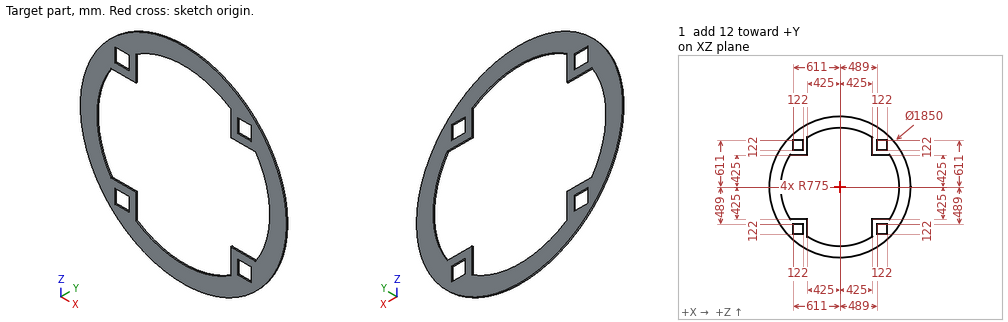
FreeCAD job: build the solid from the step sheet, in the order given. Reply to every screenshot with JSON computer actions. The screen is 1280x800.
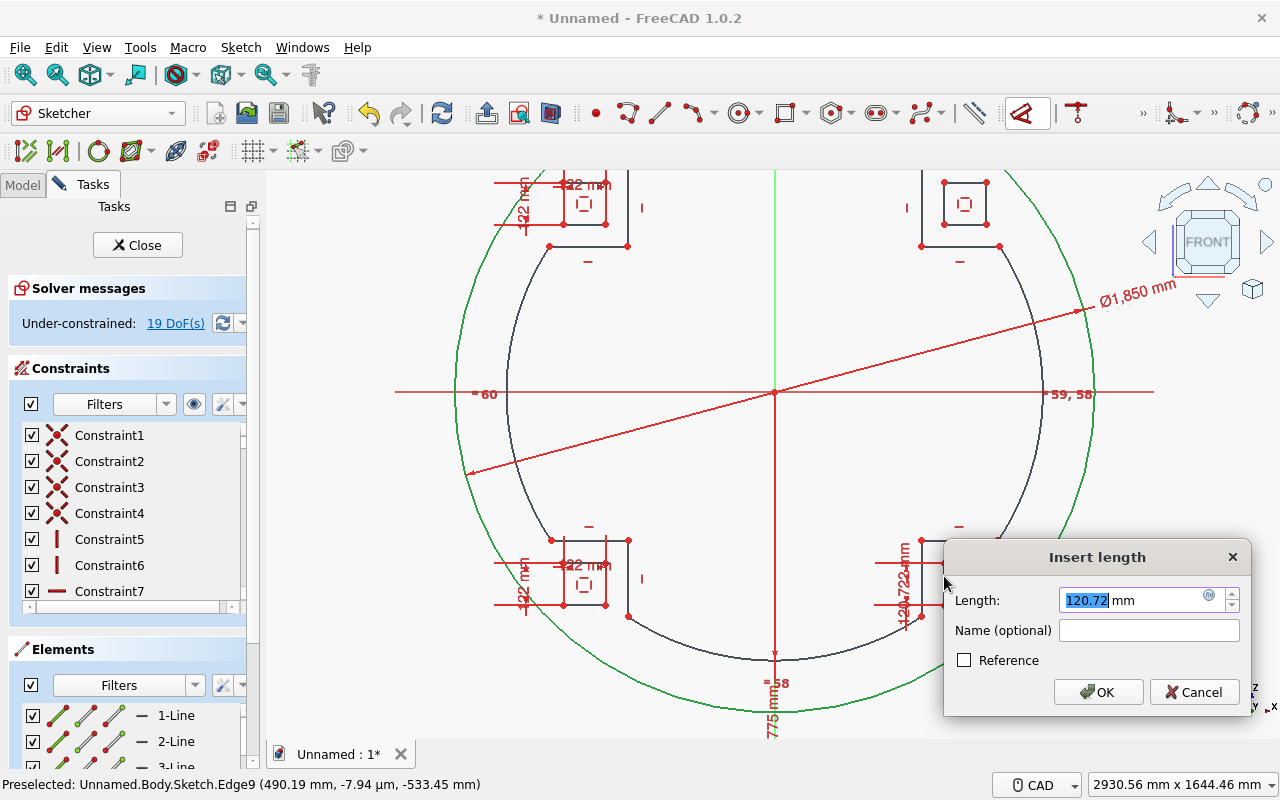
{"action": "type", "text": "122"}
{"action": "key", "text": "Return"}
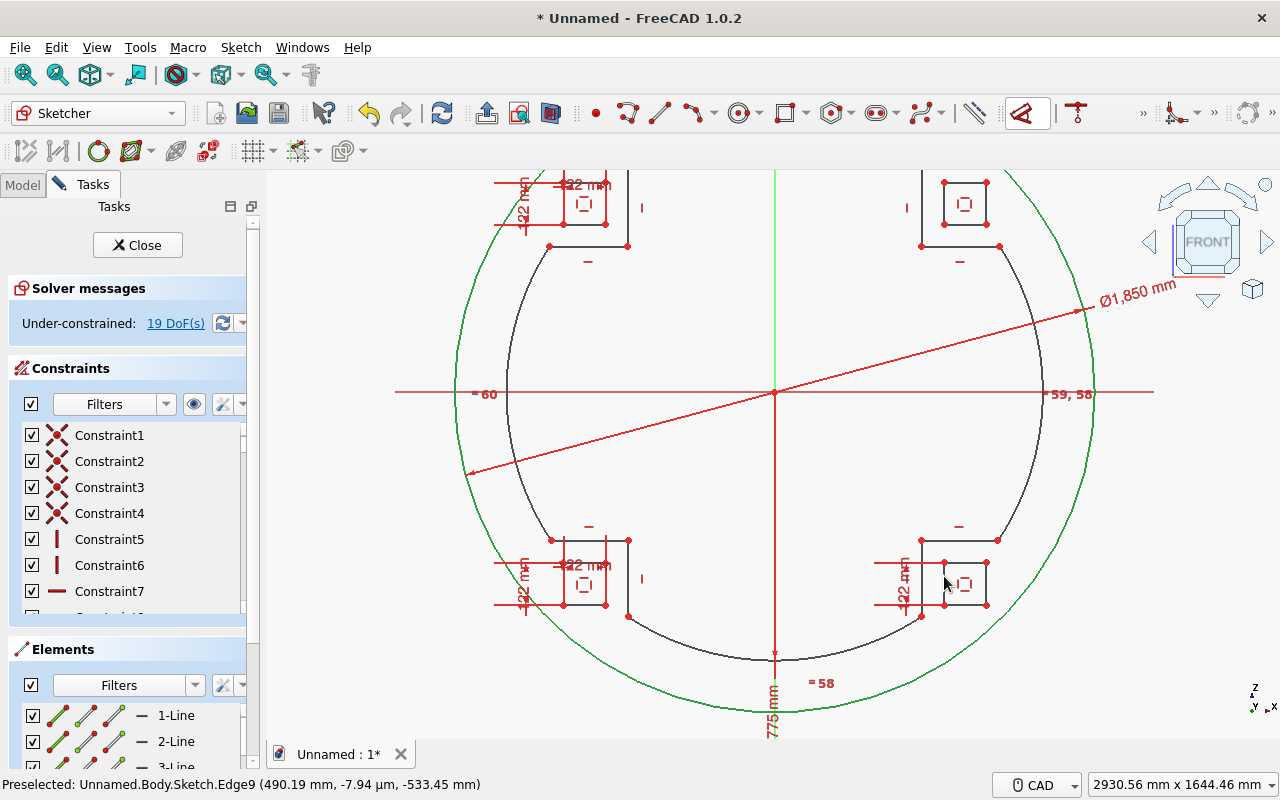
{"action": "left_click", "coordinate": [957, 605]}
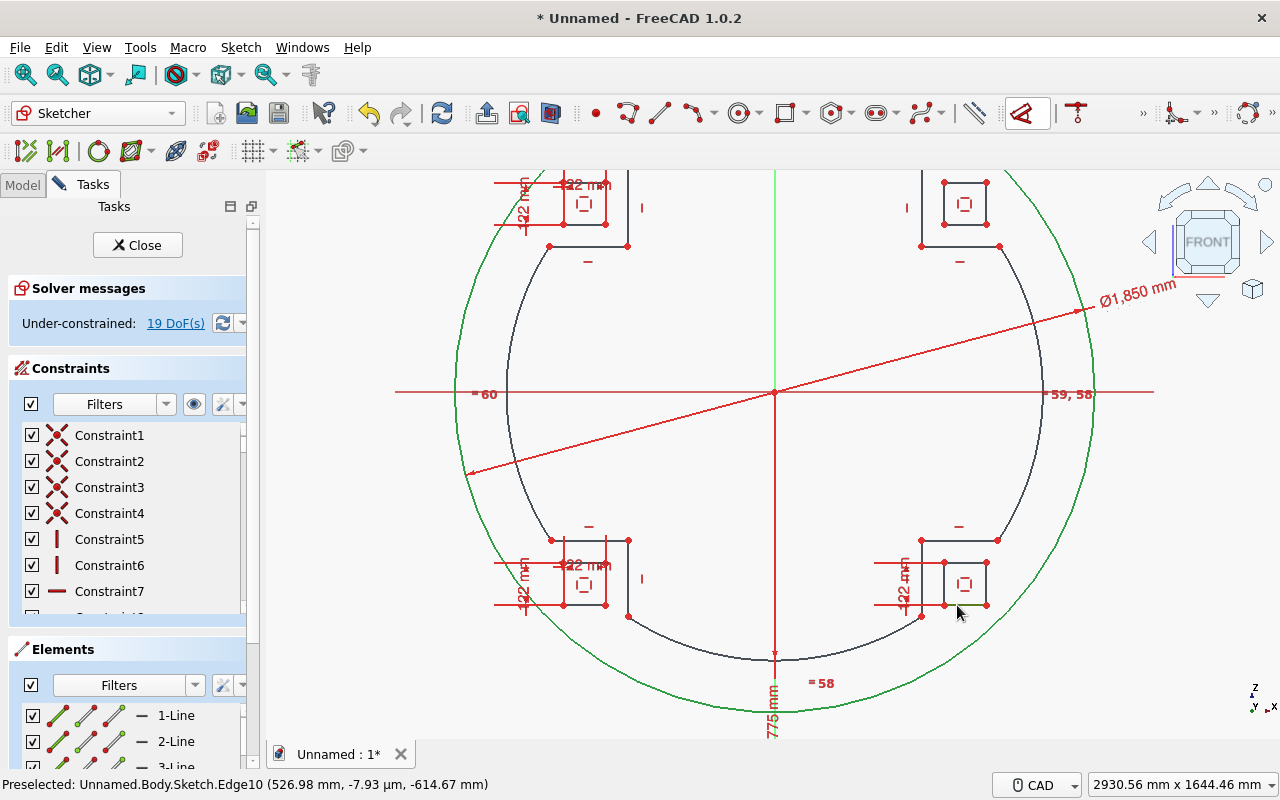
{"action": "left_click", "coordinate": [1044, 114]}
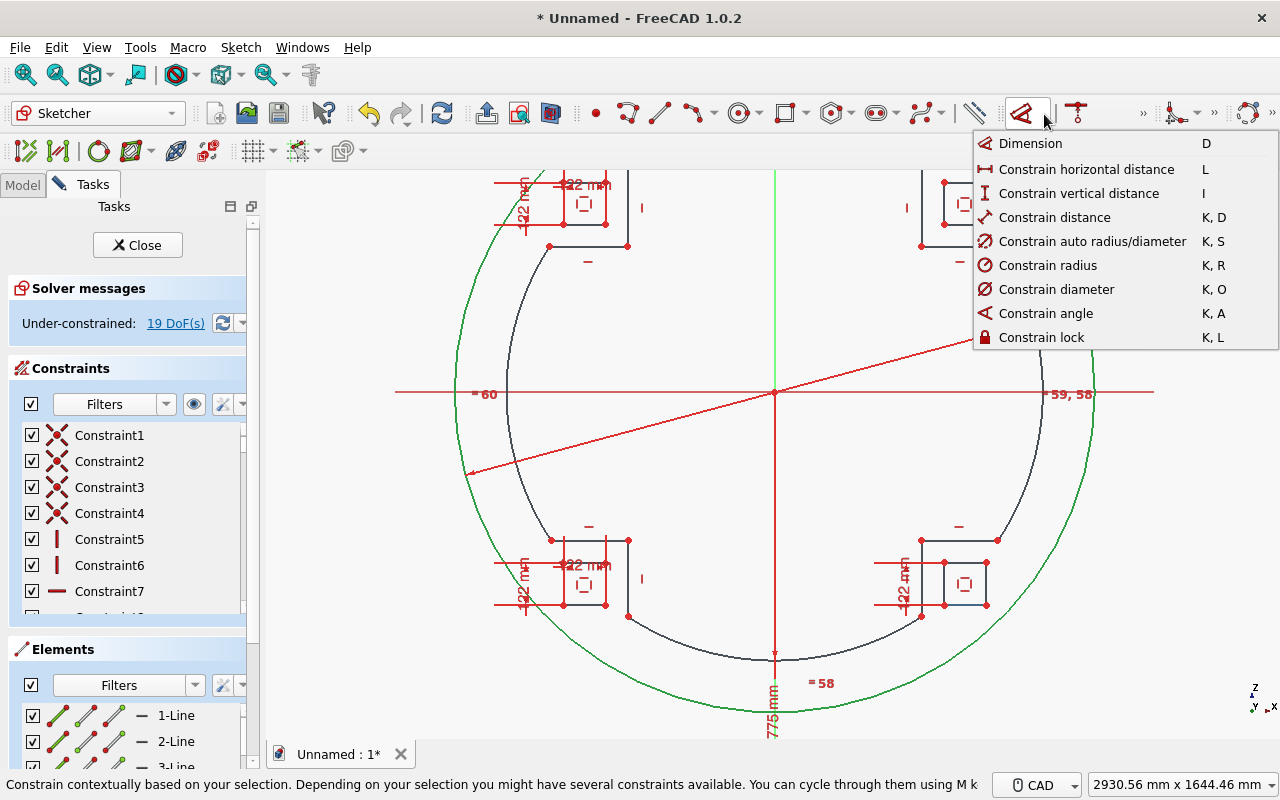
{"action": "left_click", "coordinate": [1126, 169]}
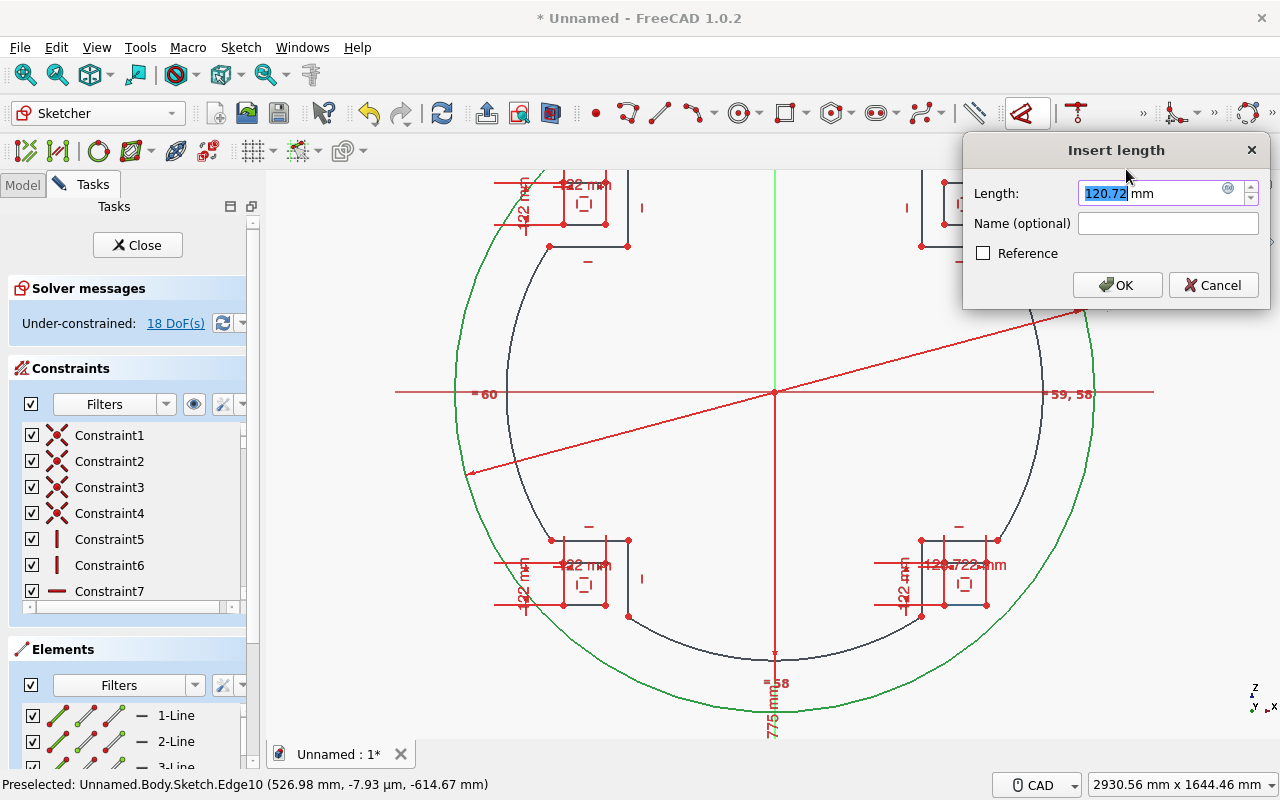
{"action": "type", "text": "122"}
{"action": "key", "text": "Return"}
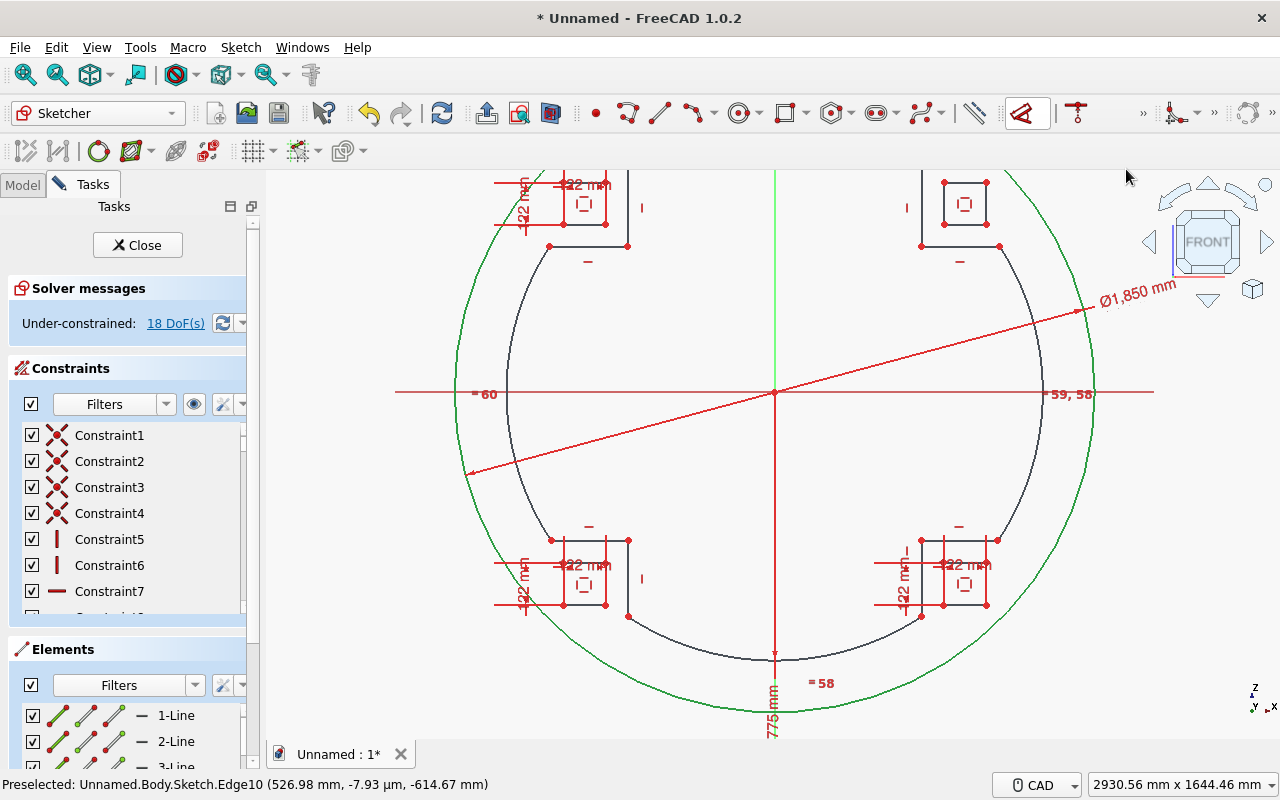
{"action": "left_click", "coordinate": [944, 212]}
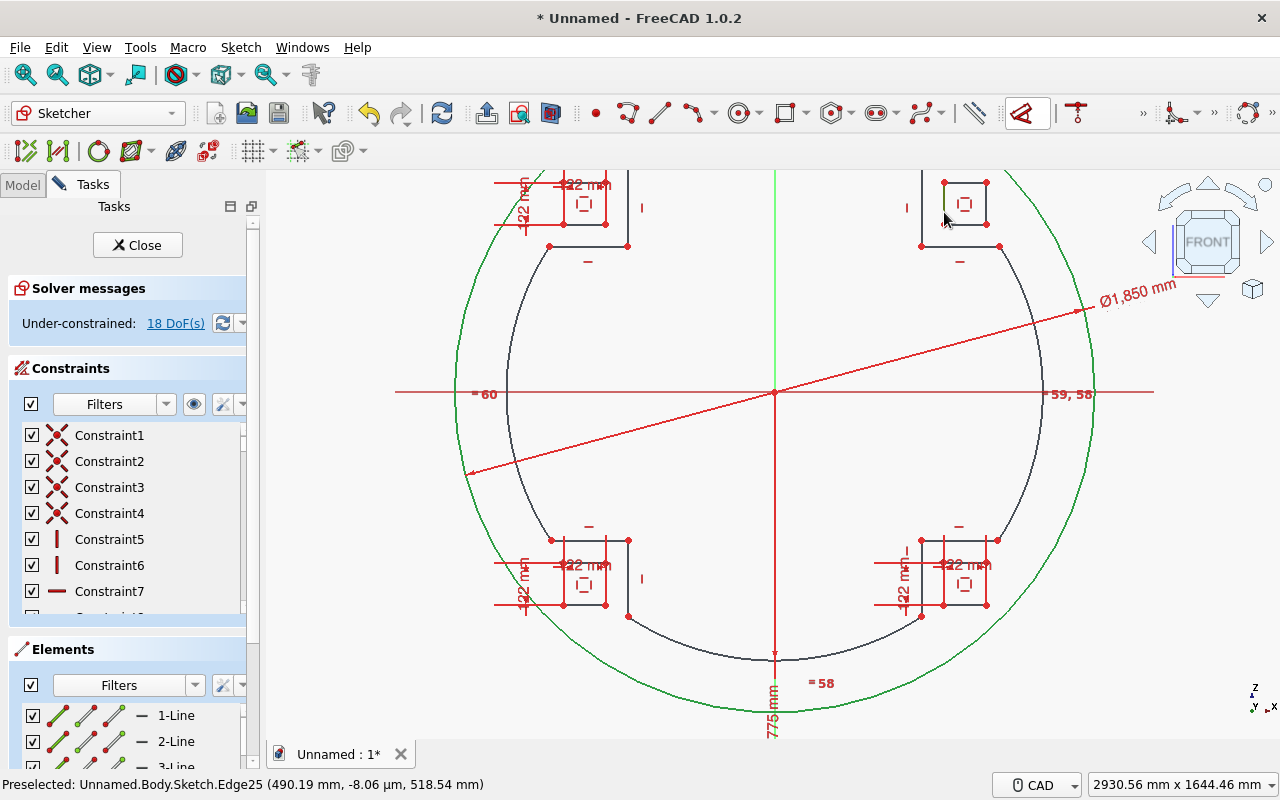
{"action": "key", "text": "i"}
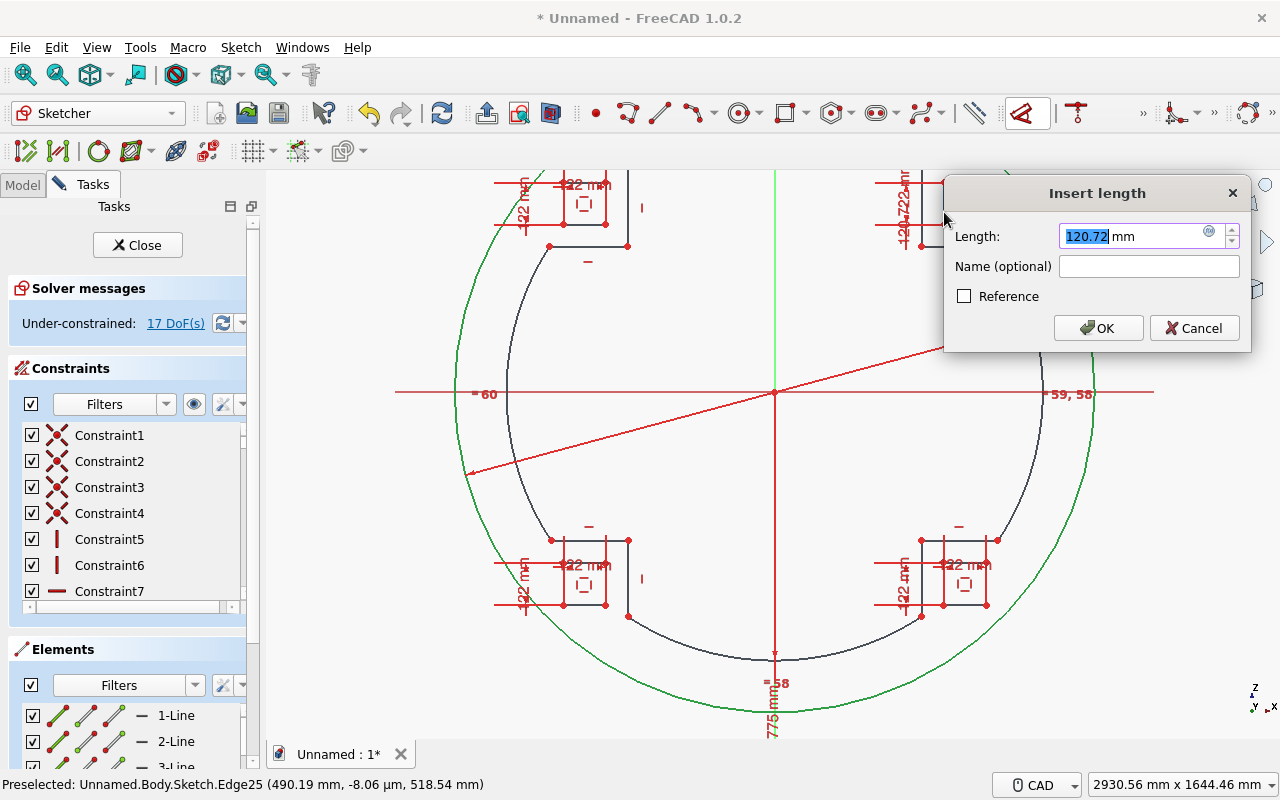
{"action": "type", "text": "122"}
{"action": "key", "text": "Return"}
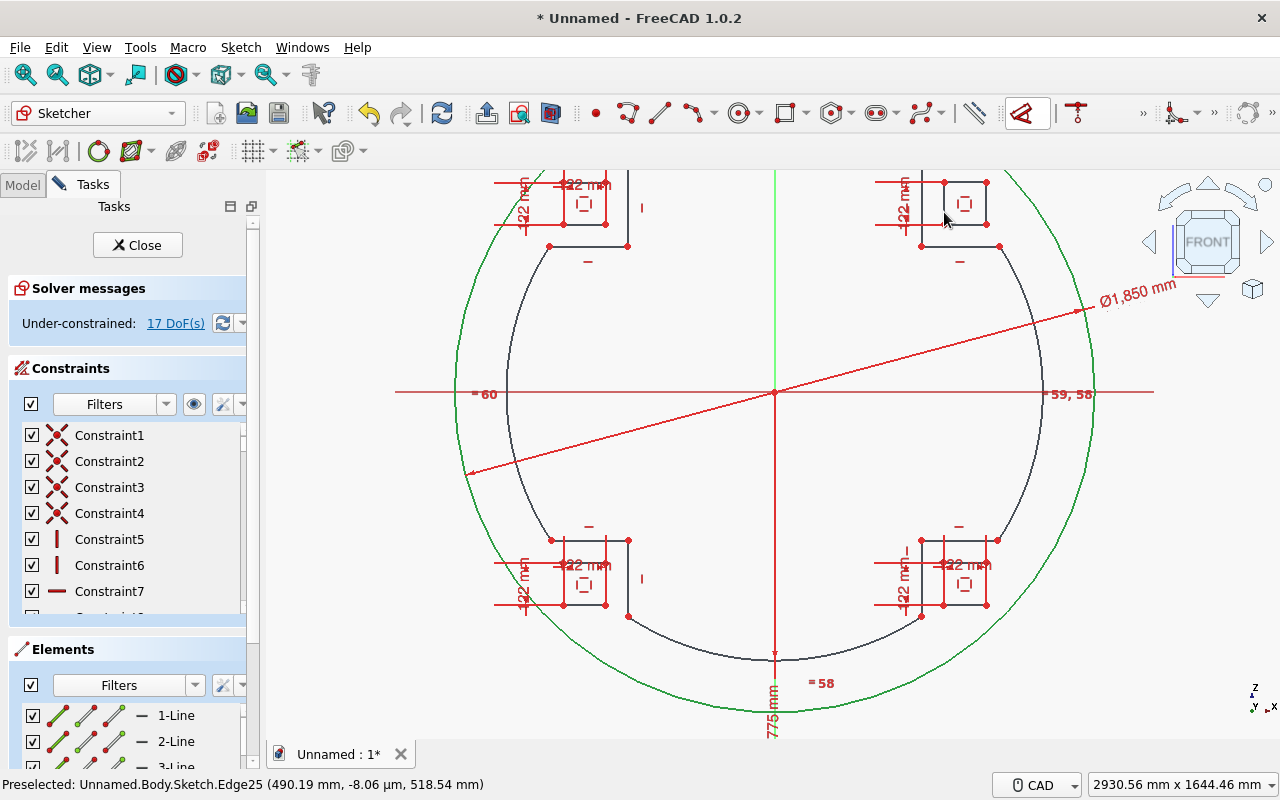
{"action": "left_click", "coordinate": [957, 225]}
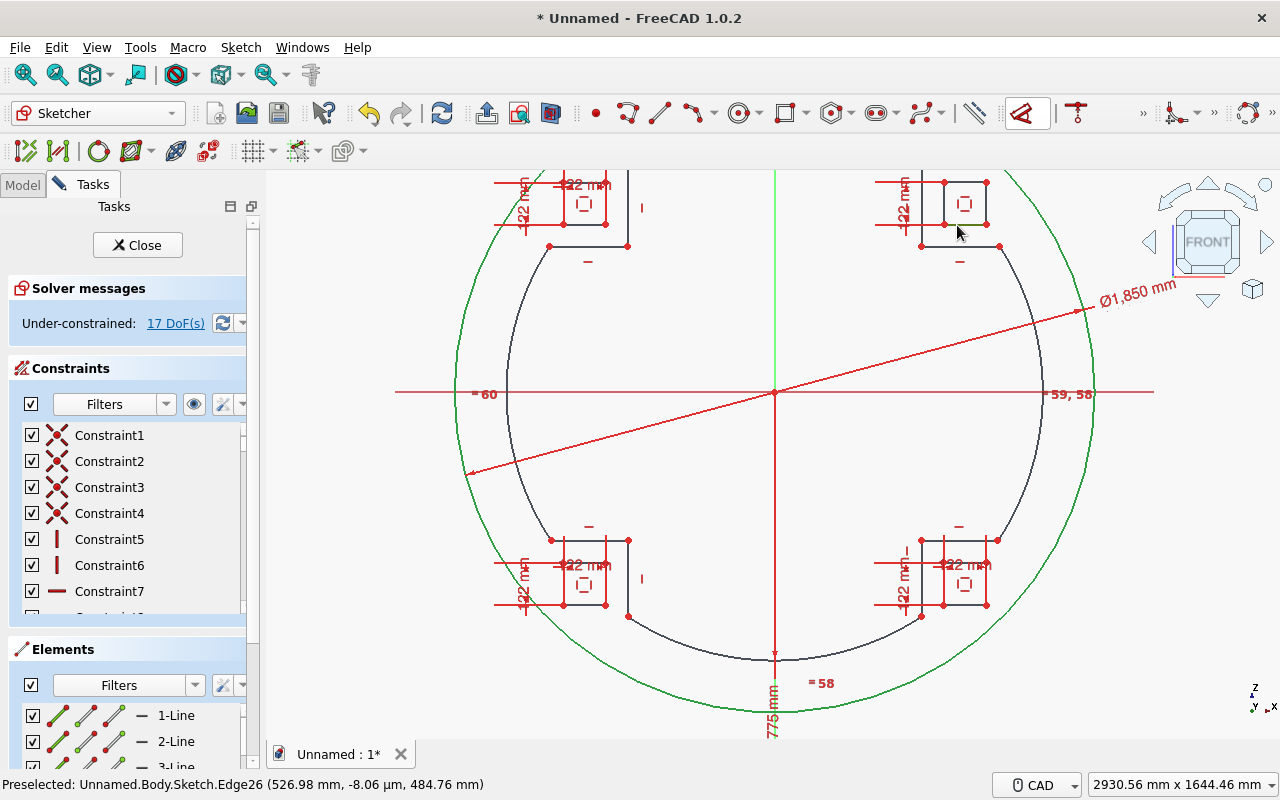
{"action": "key", "text": "l"}